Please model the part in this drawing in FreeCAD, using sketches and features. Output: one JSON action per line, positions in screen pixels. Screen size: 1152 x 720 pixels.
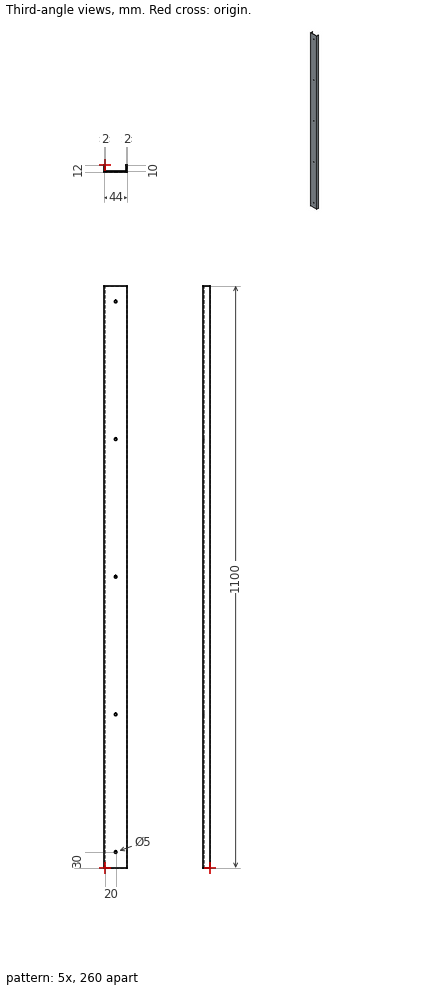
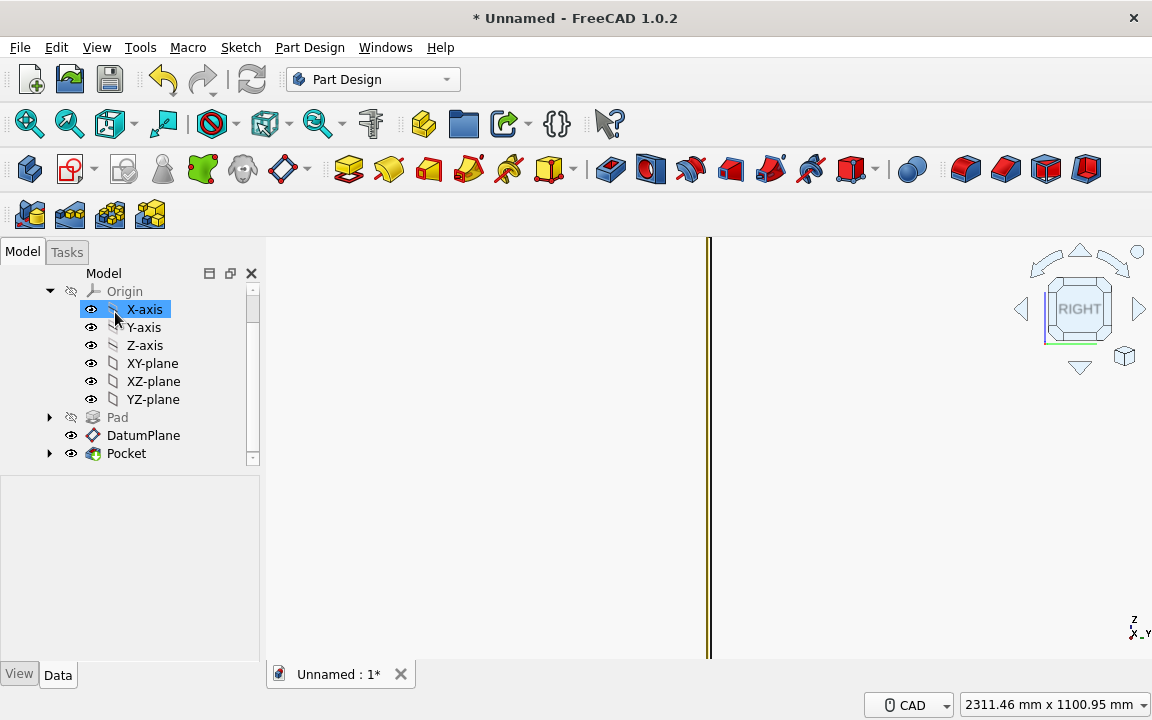
{"action": "left_click", "coordinate": [116, 435]}
{"action": "key", "text": "space"}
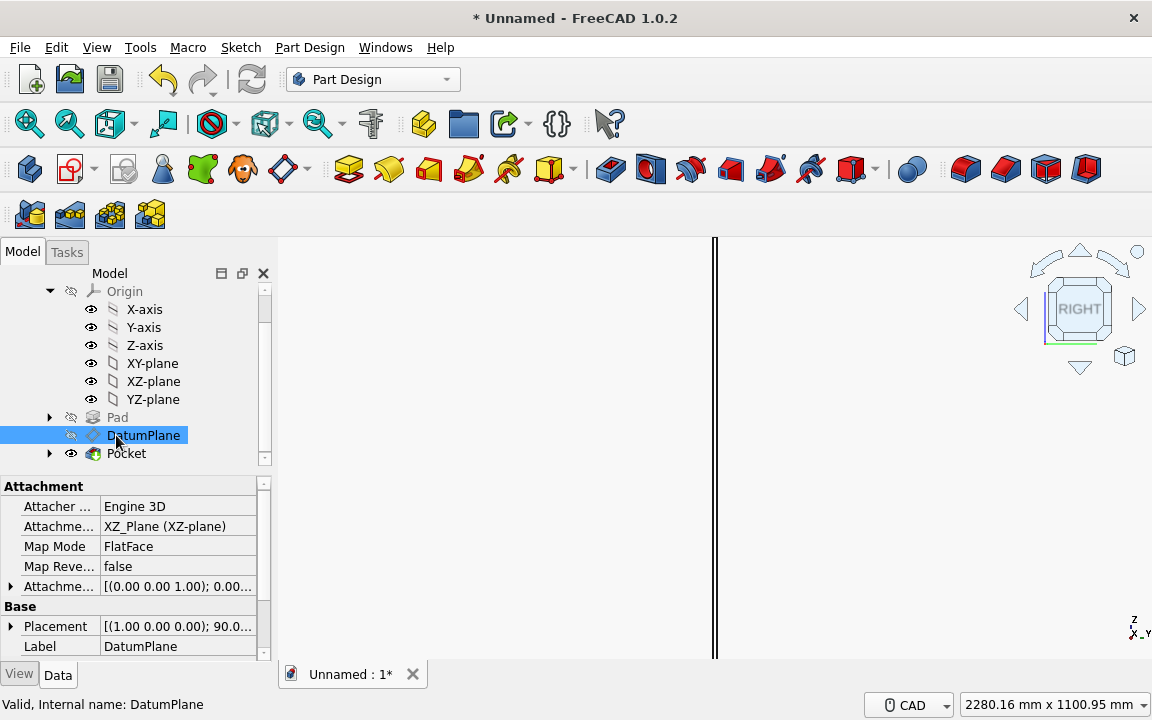
{"action": "left_click", "coordinate": [30, 124]}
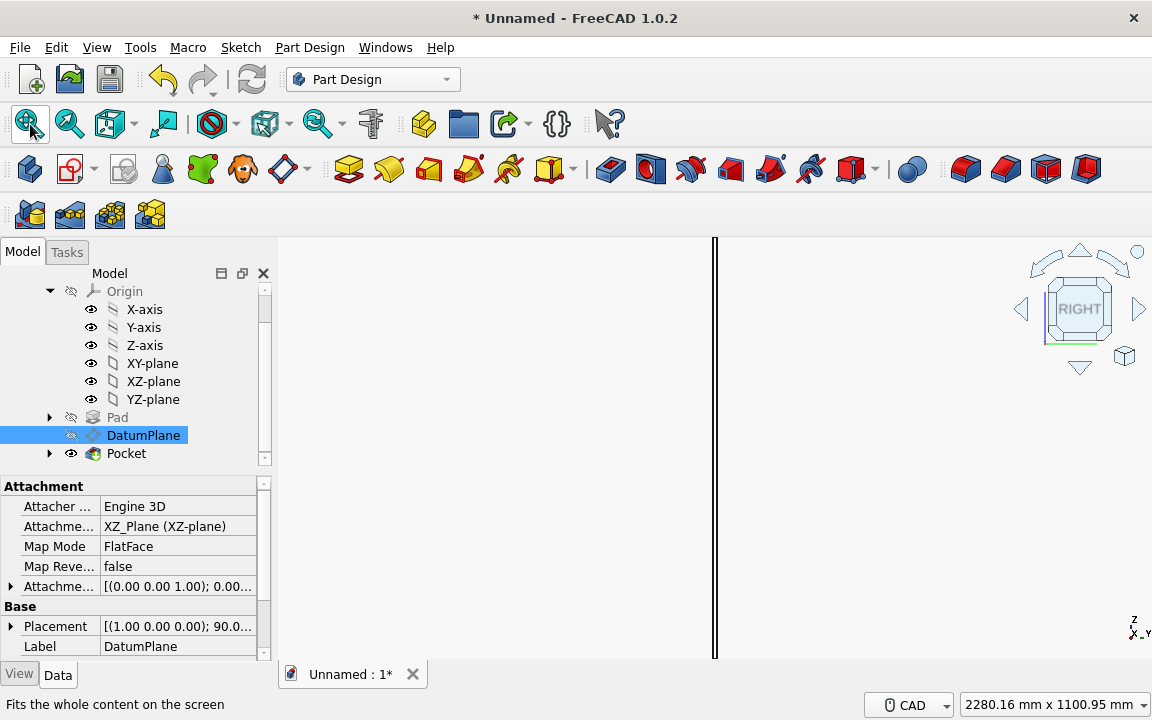
{"action": "left_click", "coordinate": [116, 453]}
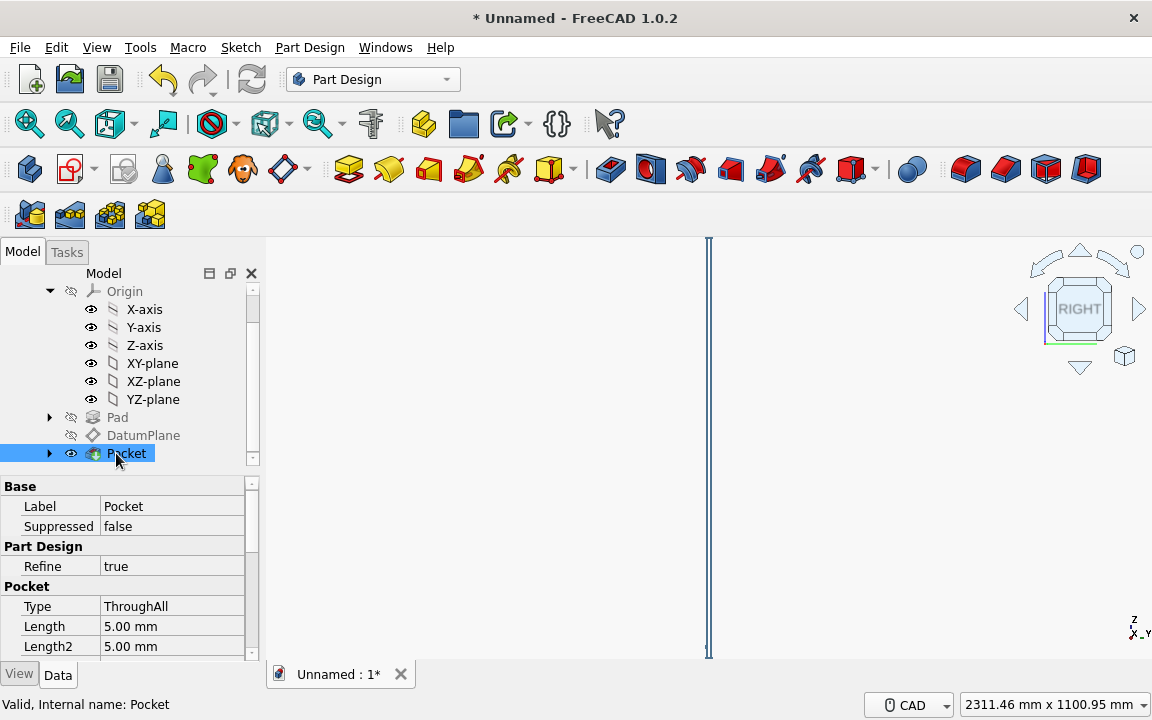
{"action": "left_click", "coordinate": [70, 214]}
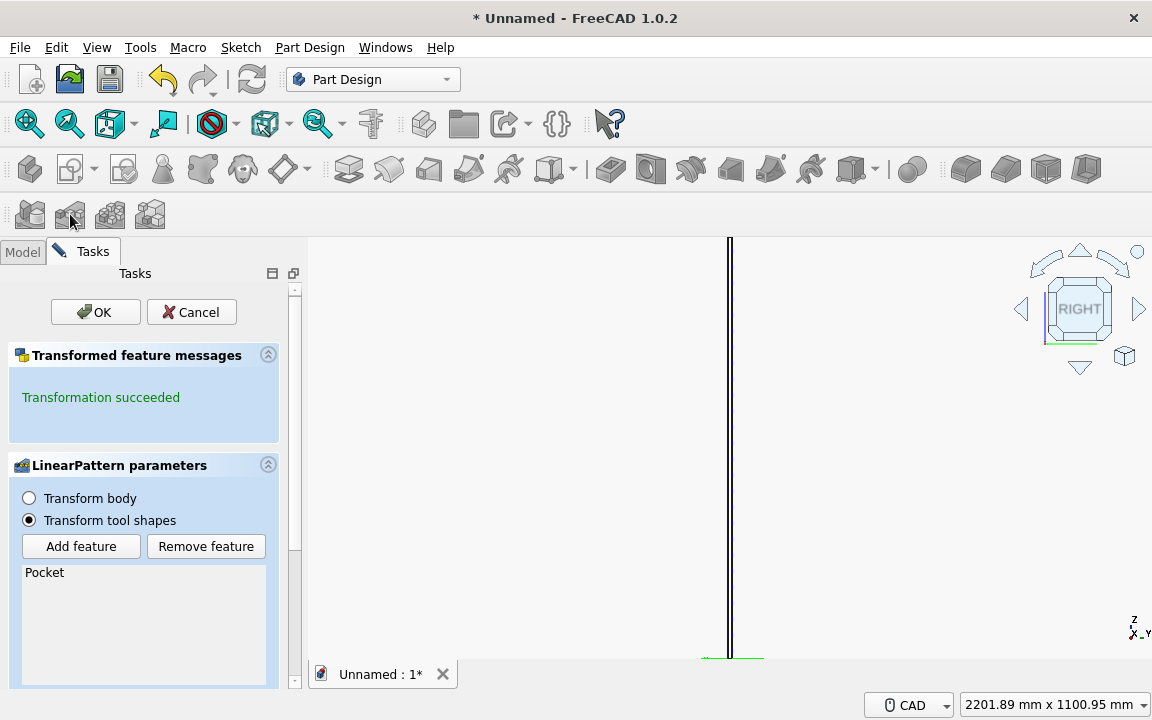
{"action": "scroll", "coordinate": [295, 486], "scroll_direction": "down", "scroll_amount": 2}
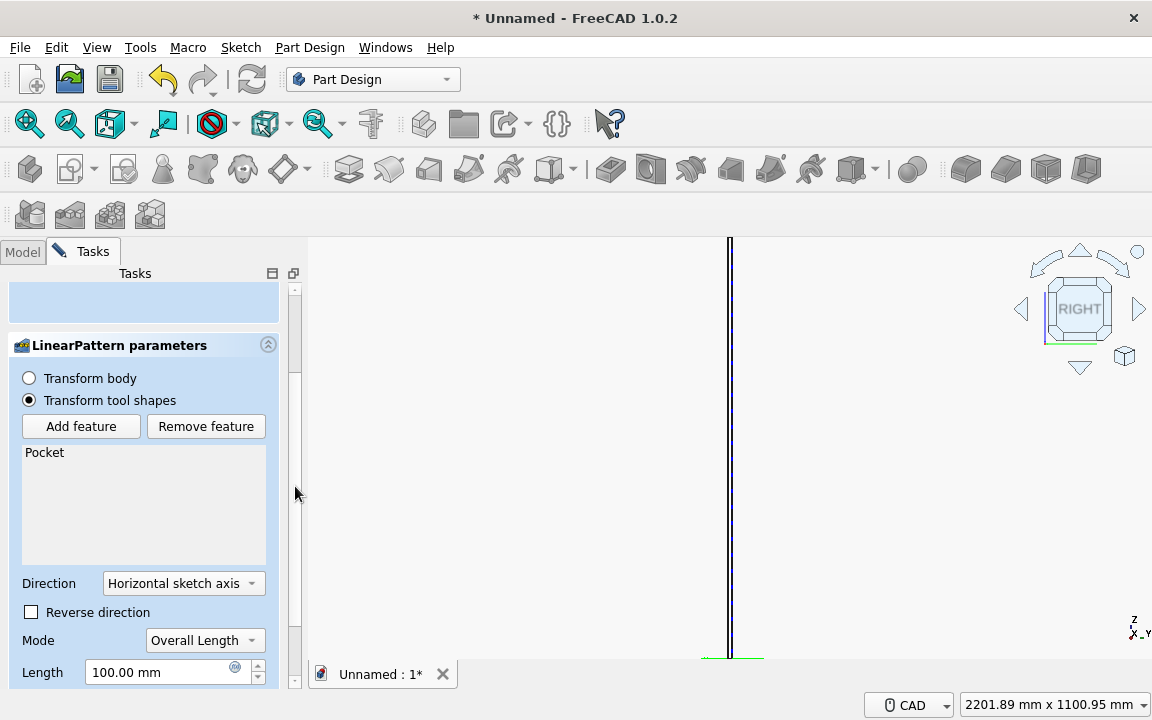
{"action": "left_click", "coordinate": [184, 584]}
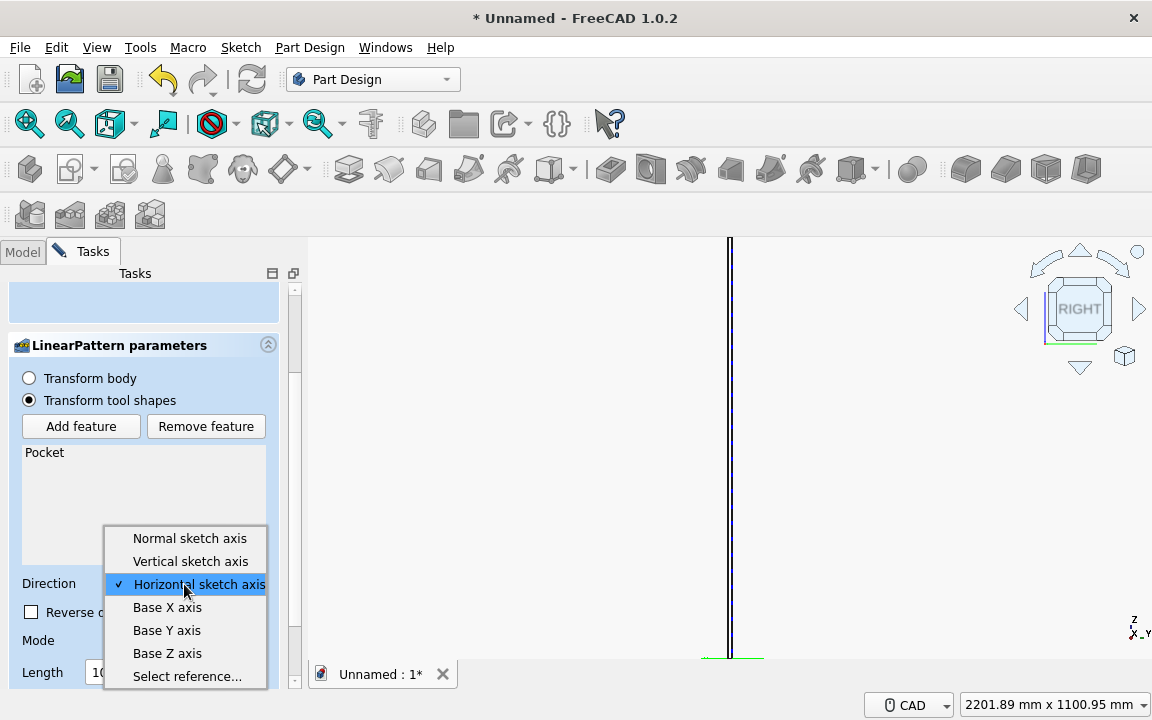
{"action": "left_click", "coordinate": [184, 654]}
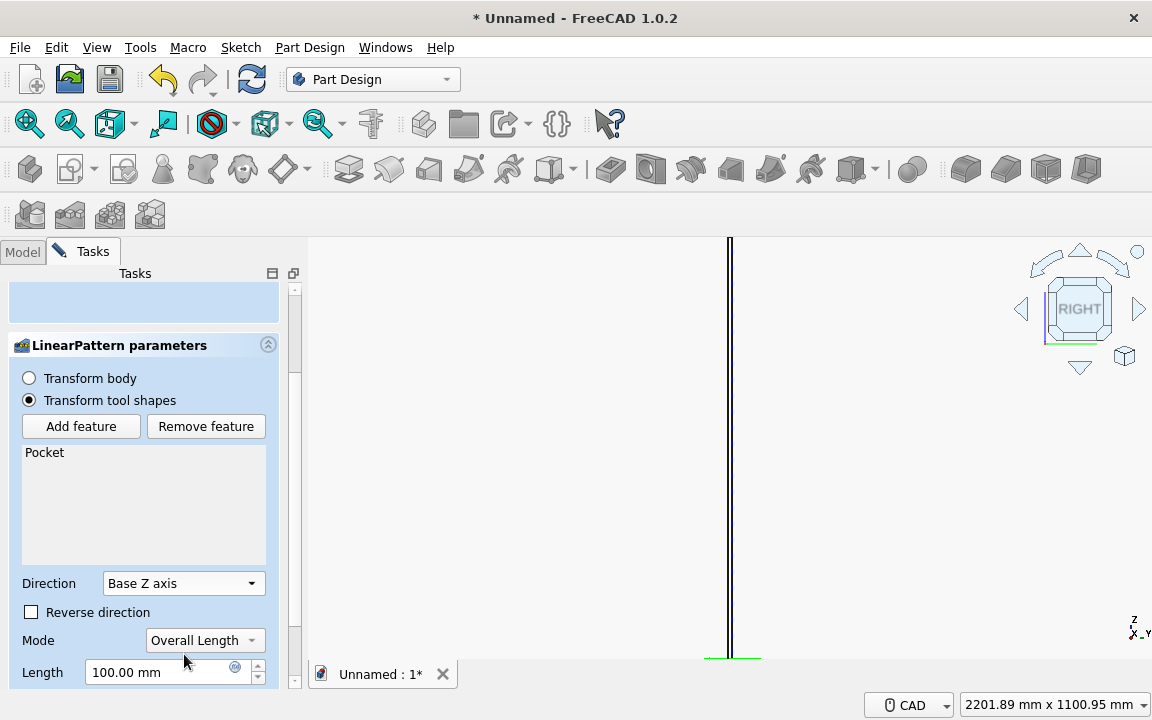
{"action": "left_click", "coordinate": [206, 640]}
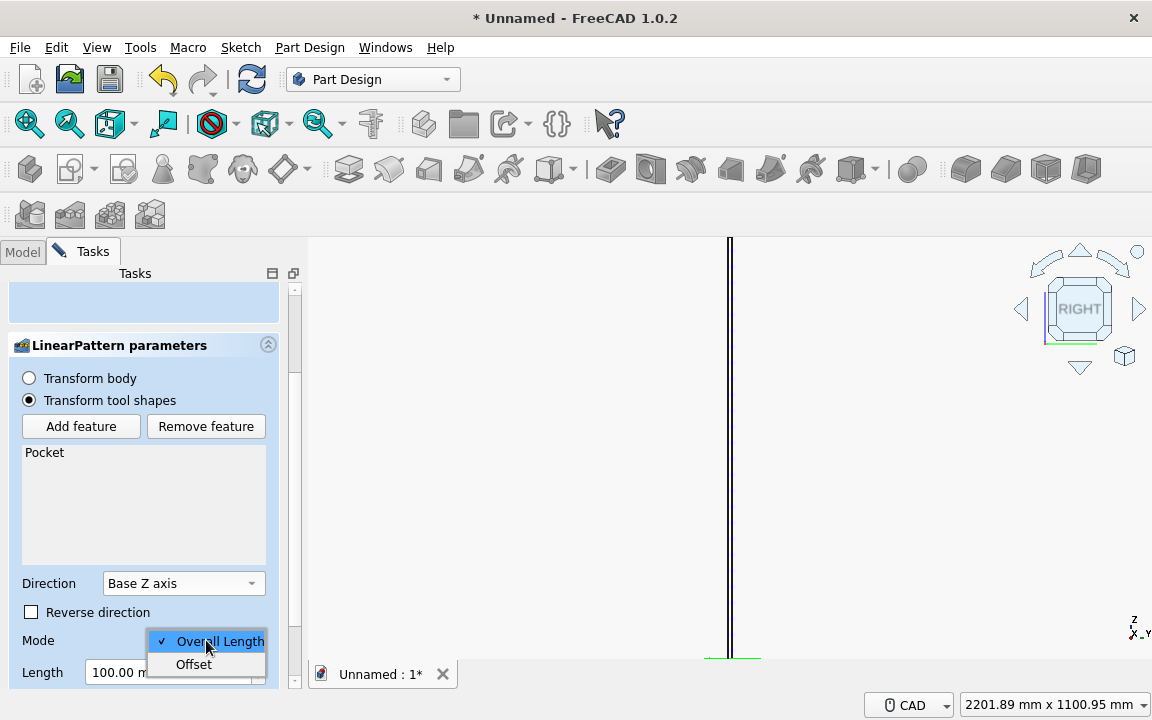
{"action": "left_click", "coordinate": [206, 664]}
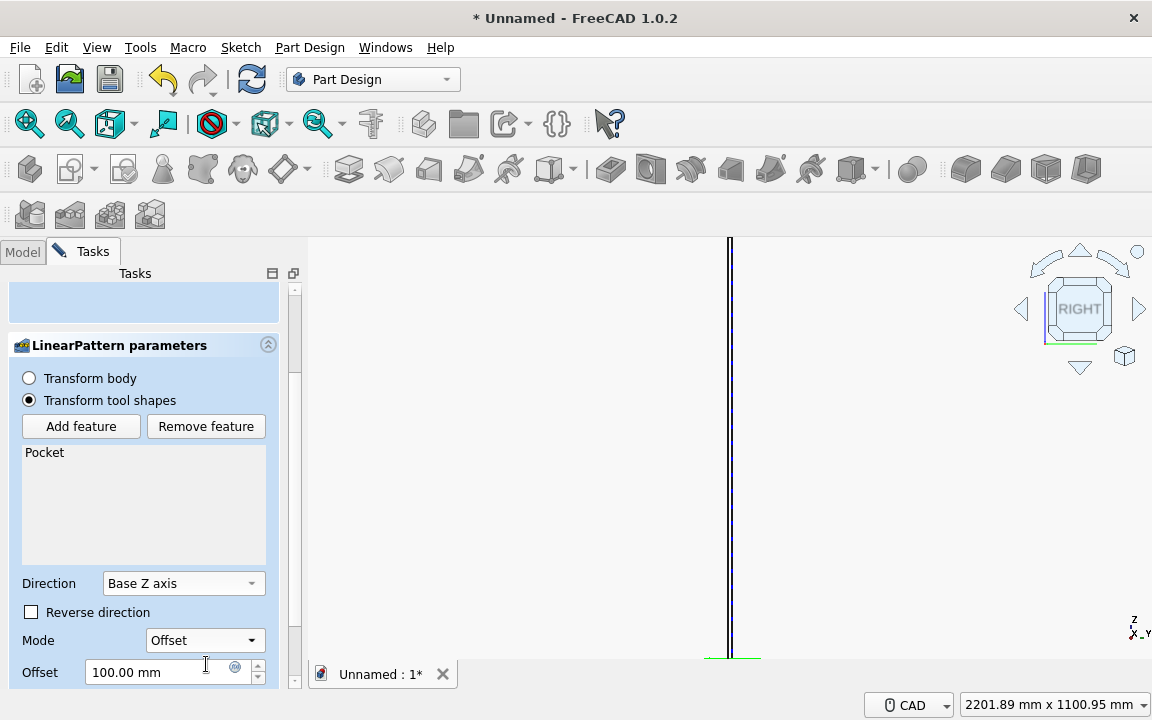
{"action": "triple_click", "coordinate": [168, 672]}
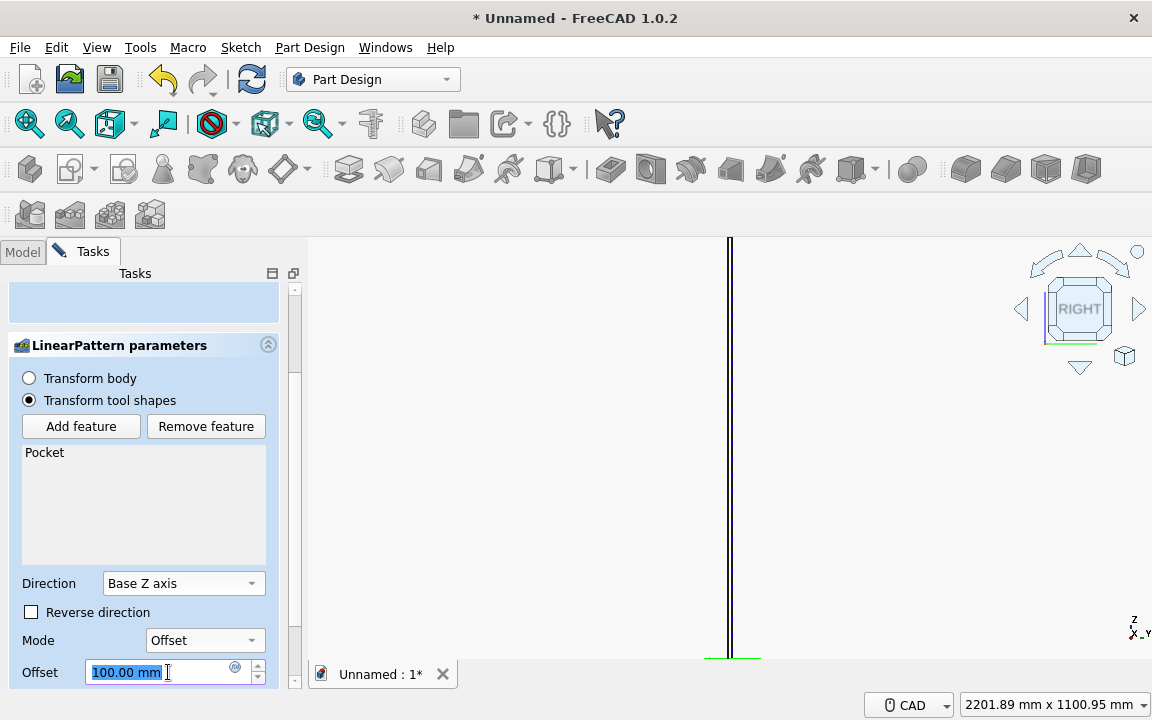
{"action": "type", "text": "260"}
{"action": "key", "text": "Tab"}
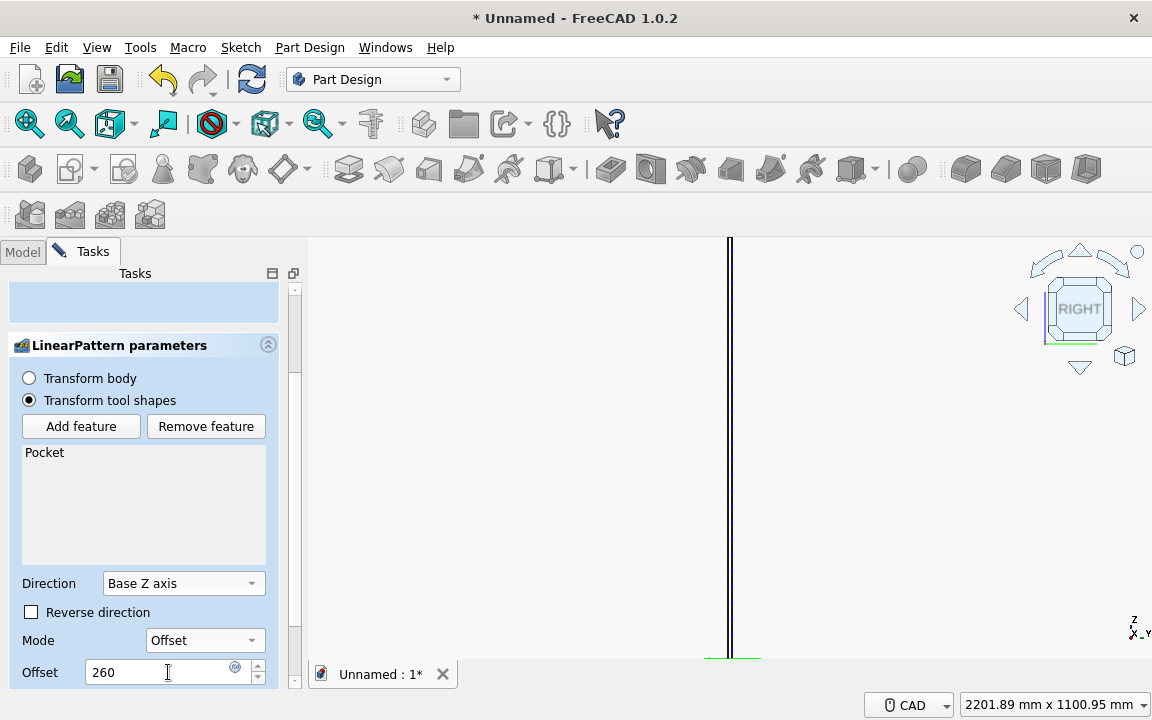
{"action": "scroll", "coordinate": [295, 486], "scroll_direction": "down", "scroll_amount": 2}